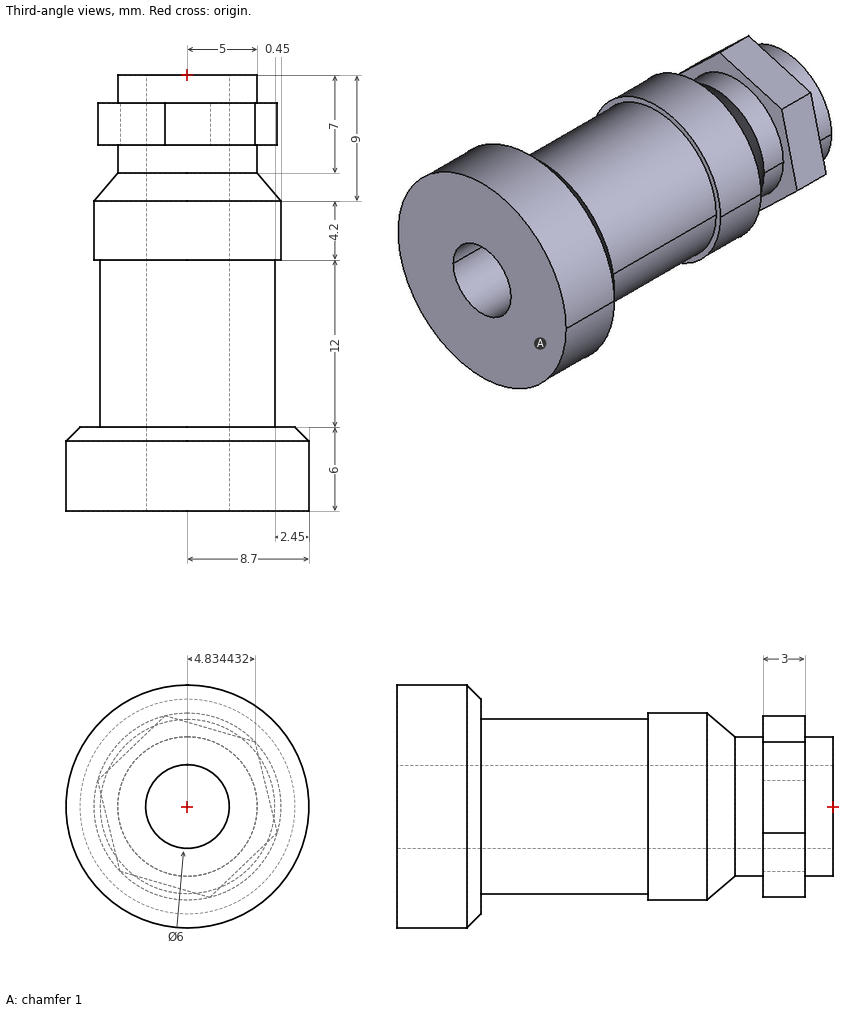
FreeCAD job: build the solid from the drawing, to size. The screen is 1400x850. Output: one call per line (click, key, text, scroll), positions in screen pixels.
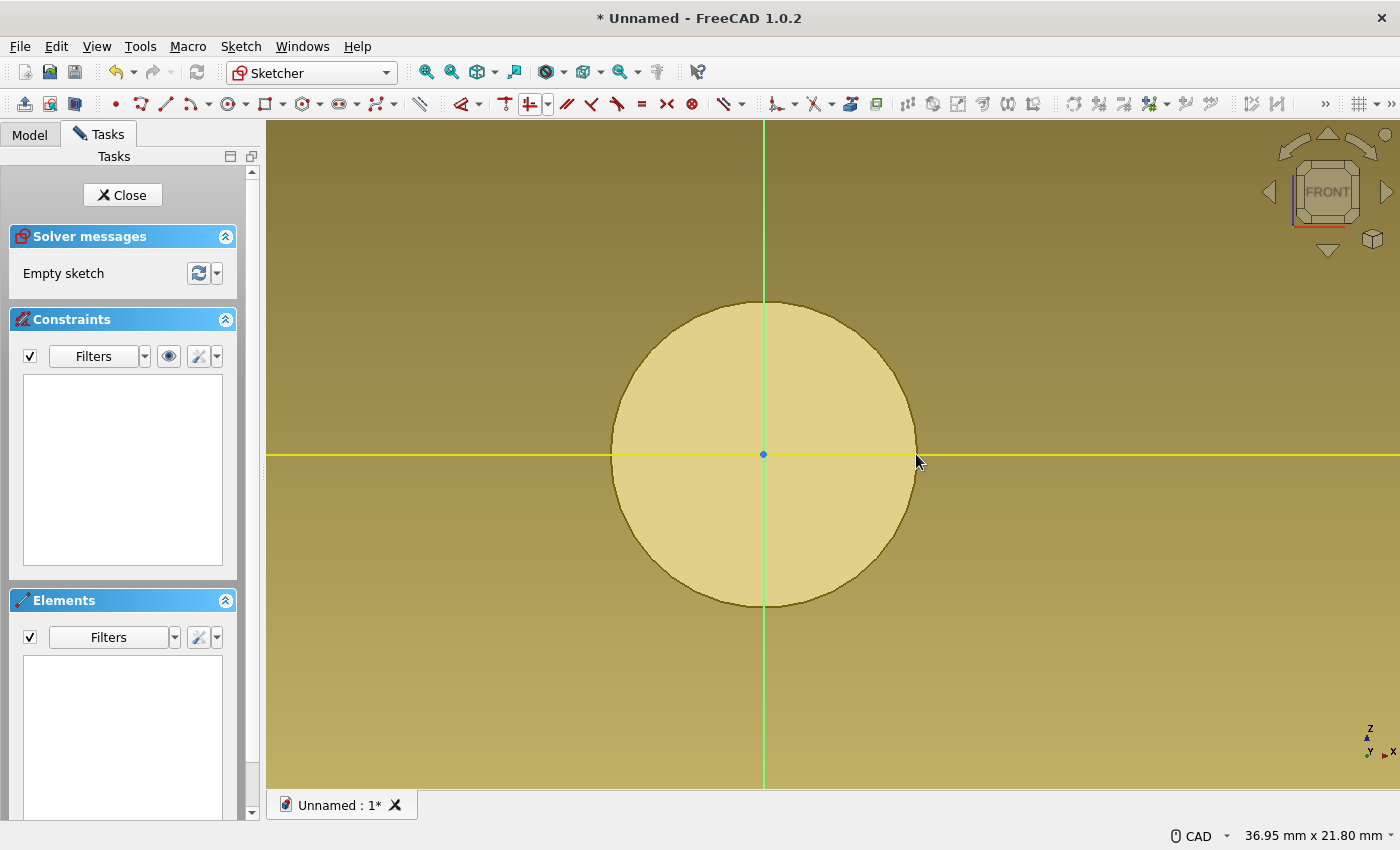
key(g)
key(p)
key(6)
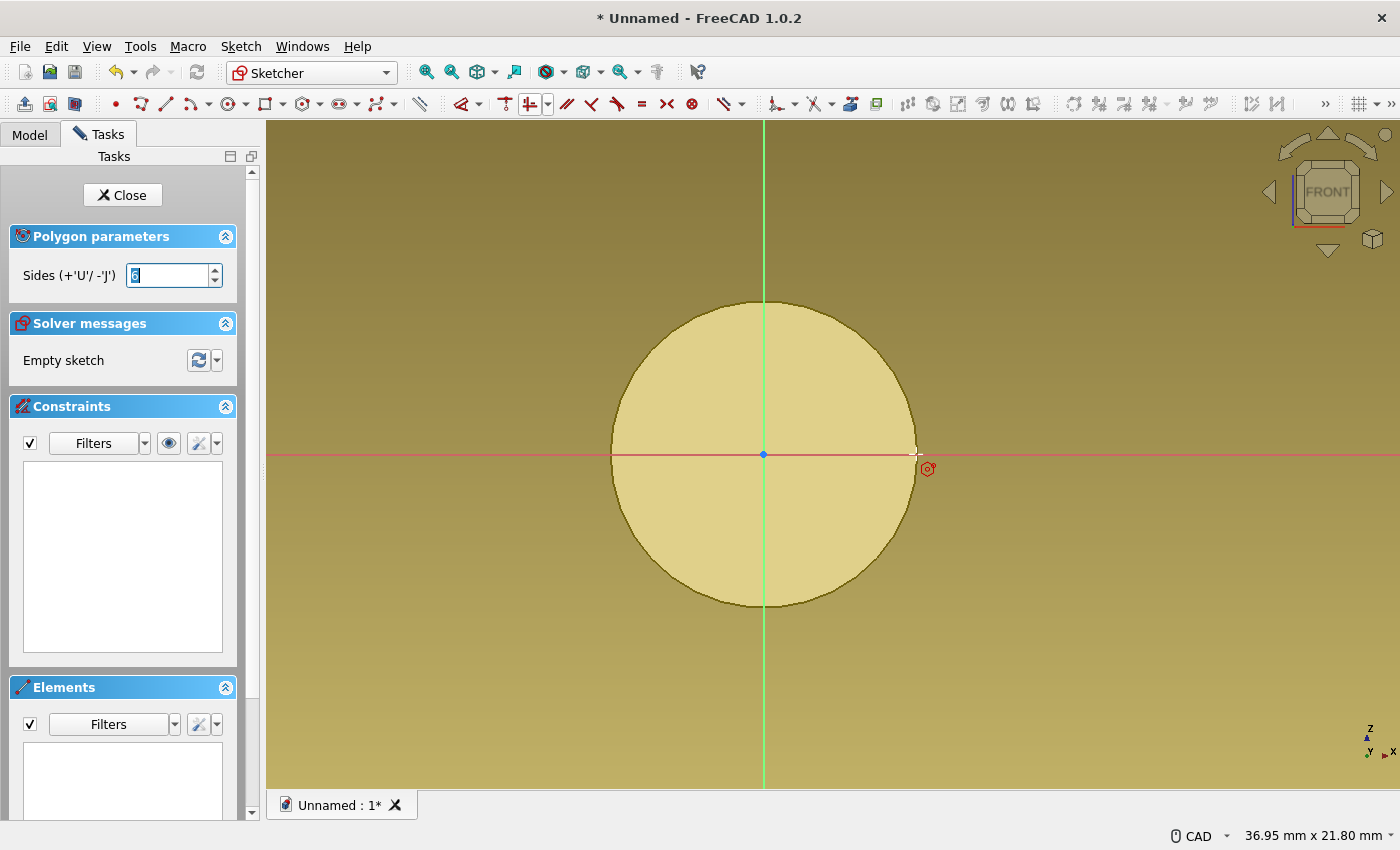
click(764, 454)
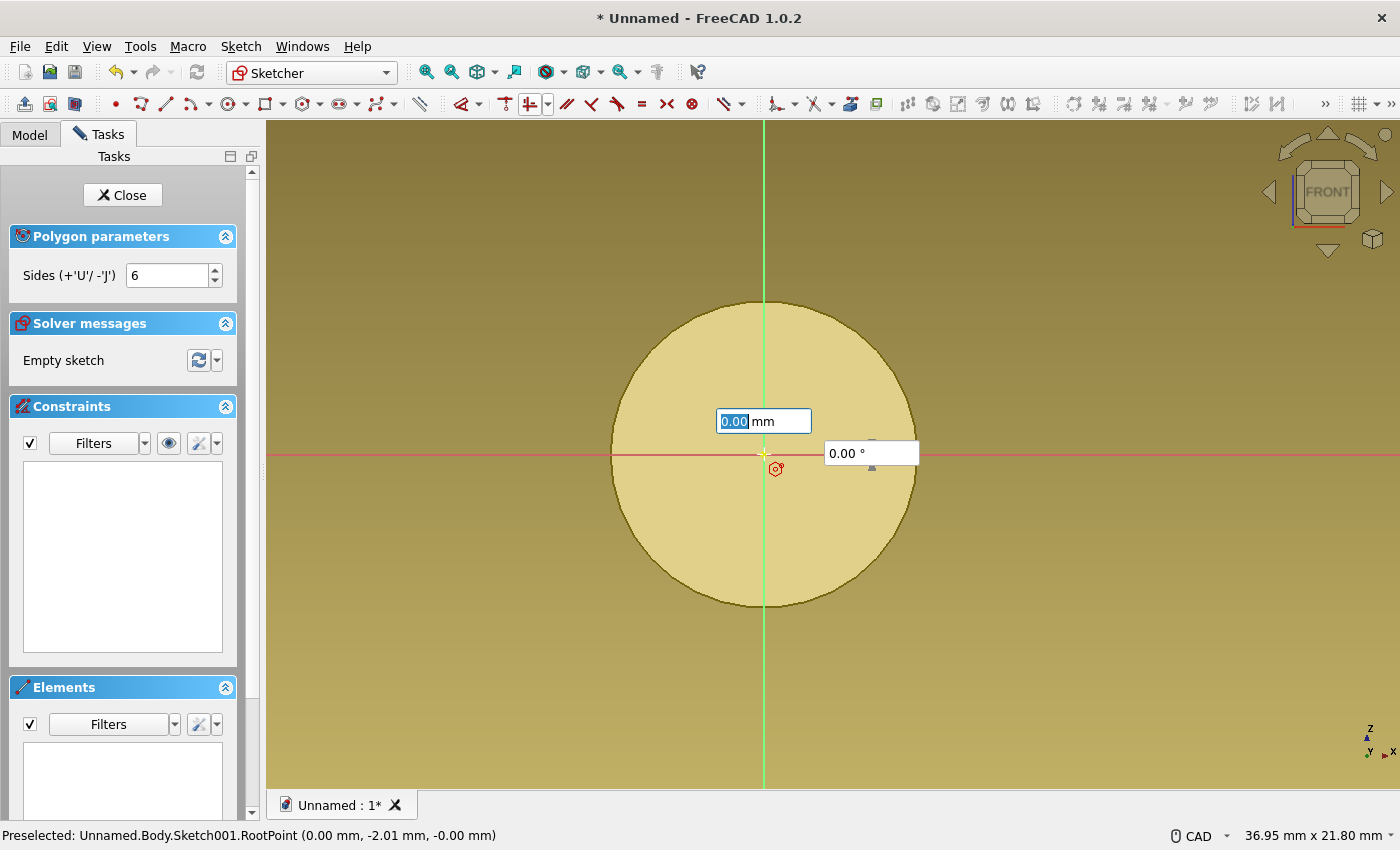
click(912, 312)
right_click(912, 312)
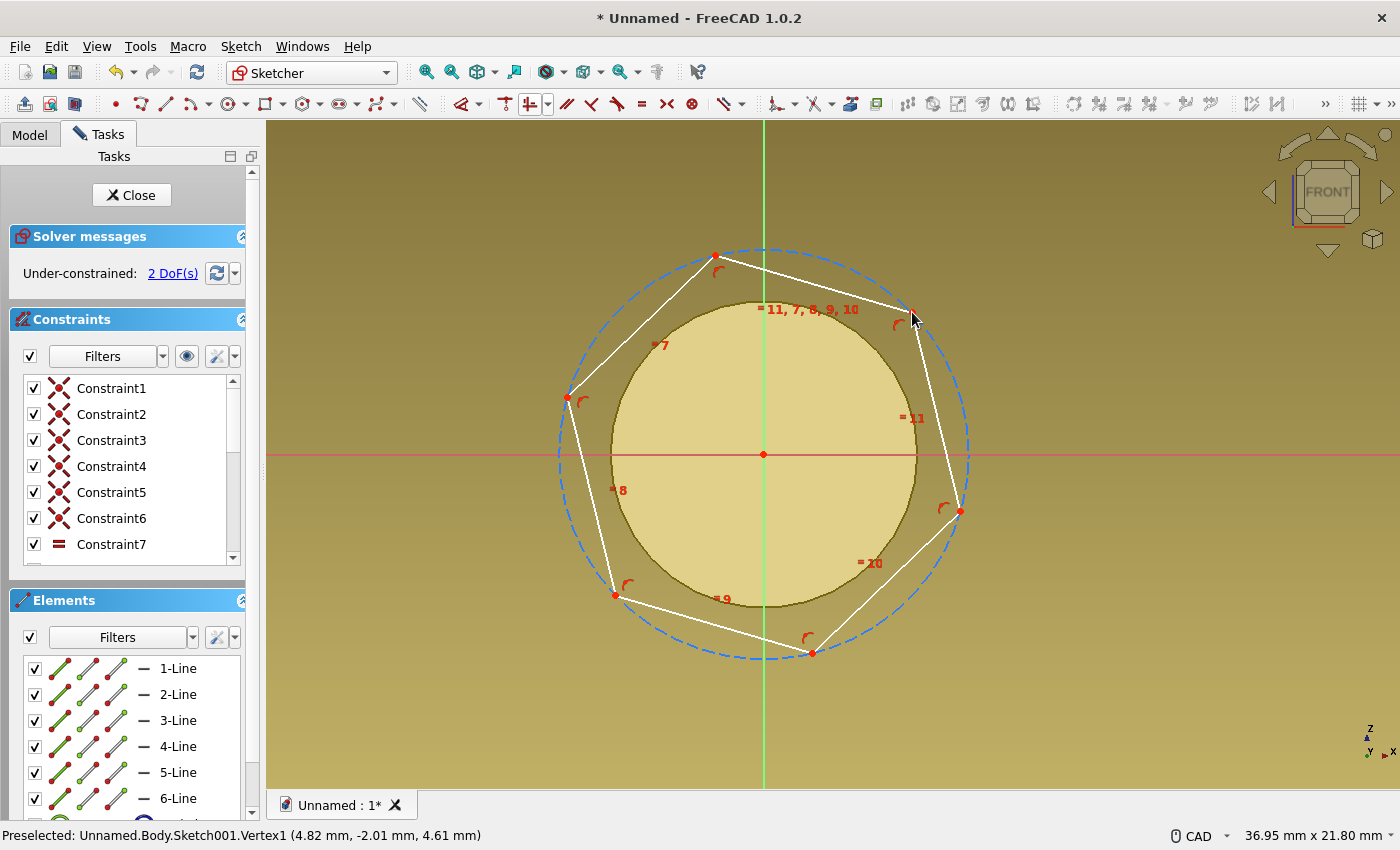
key(d)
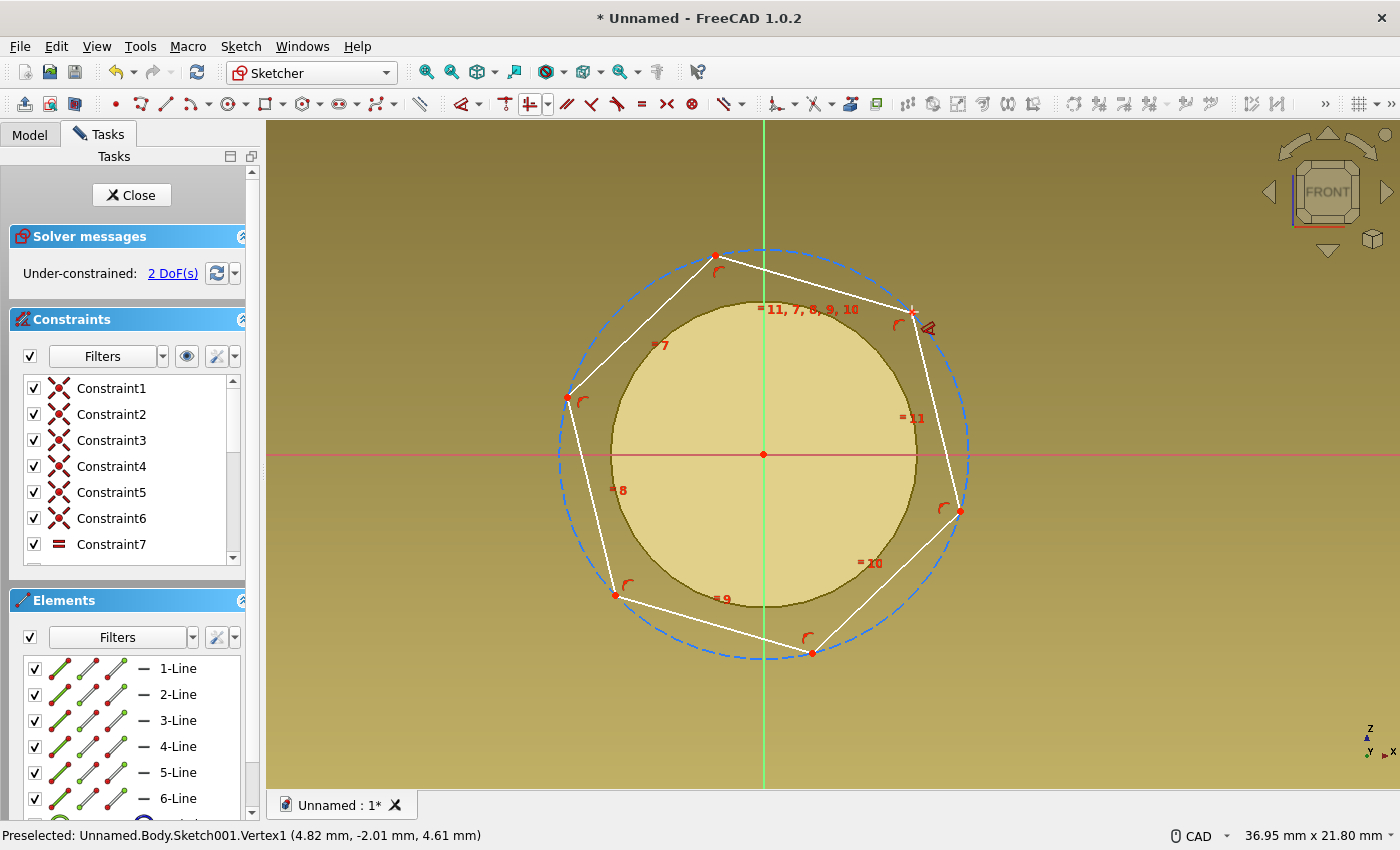
click(619, 310)
click(596, 287)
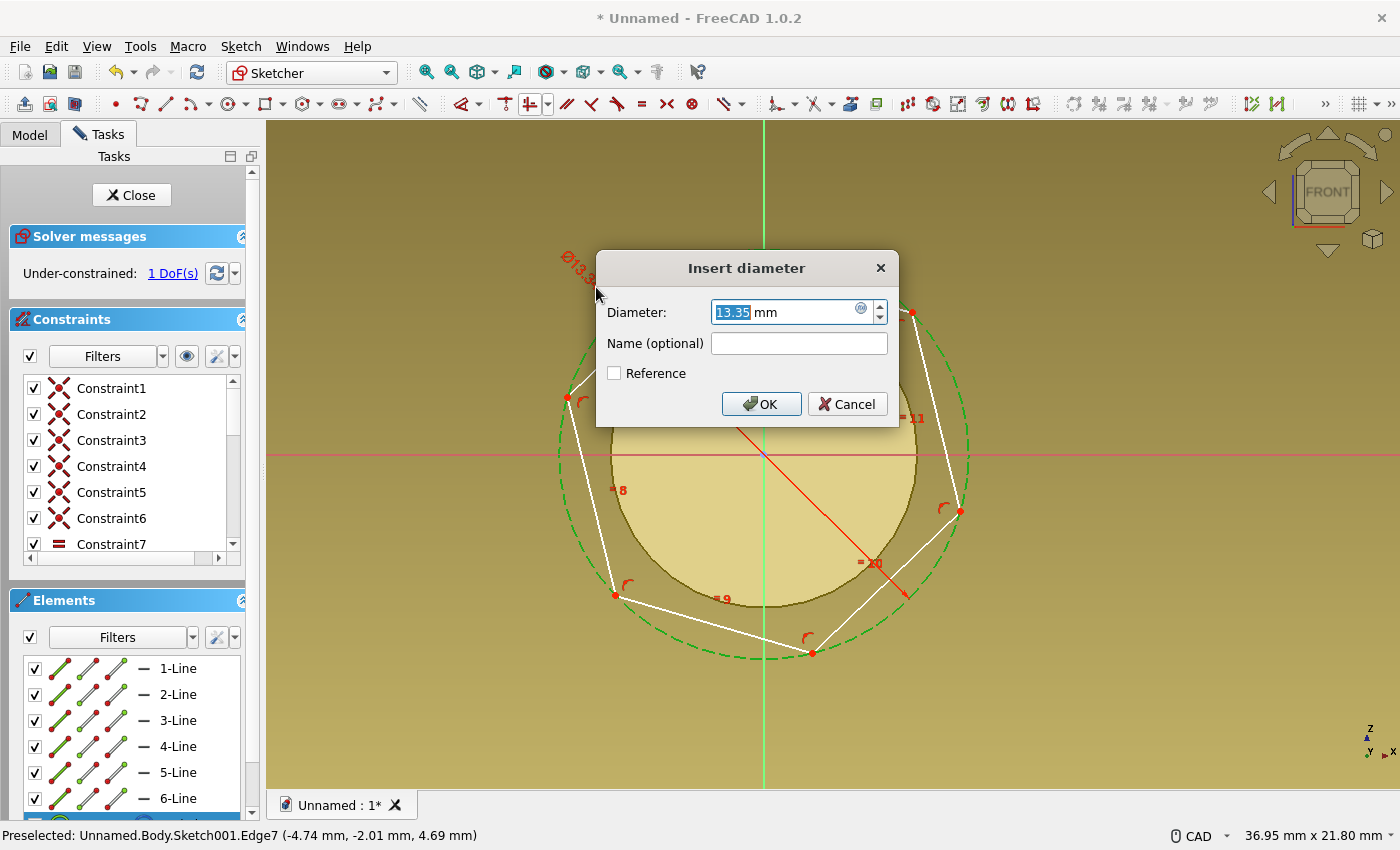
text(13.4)
key(Return)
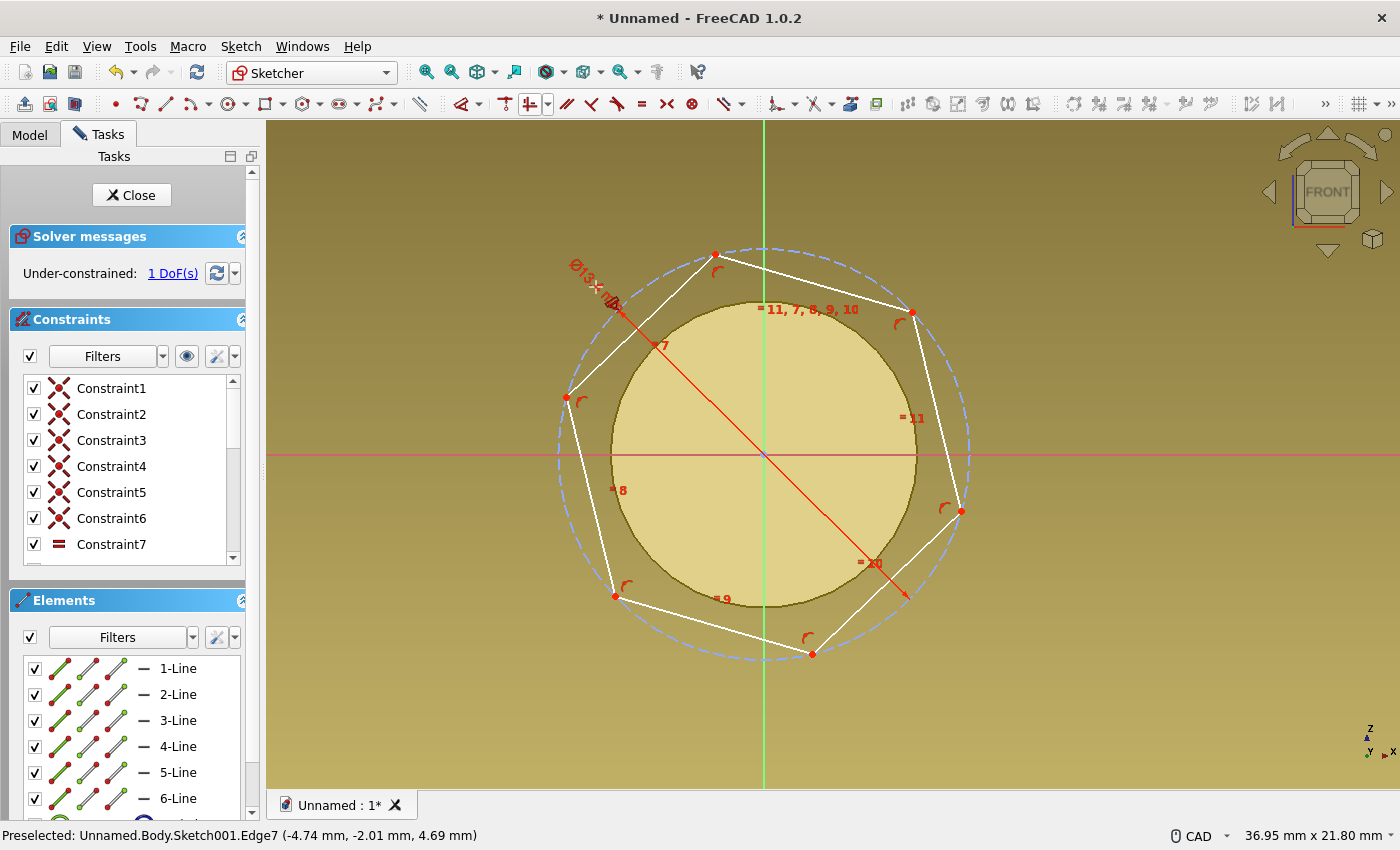
click(912, 312)
click(838, 488)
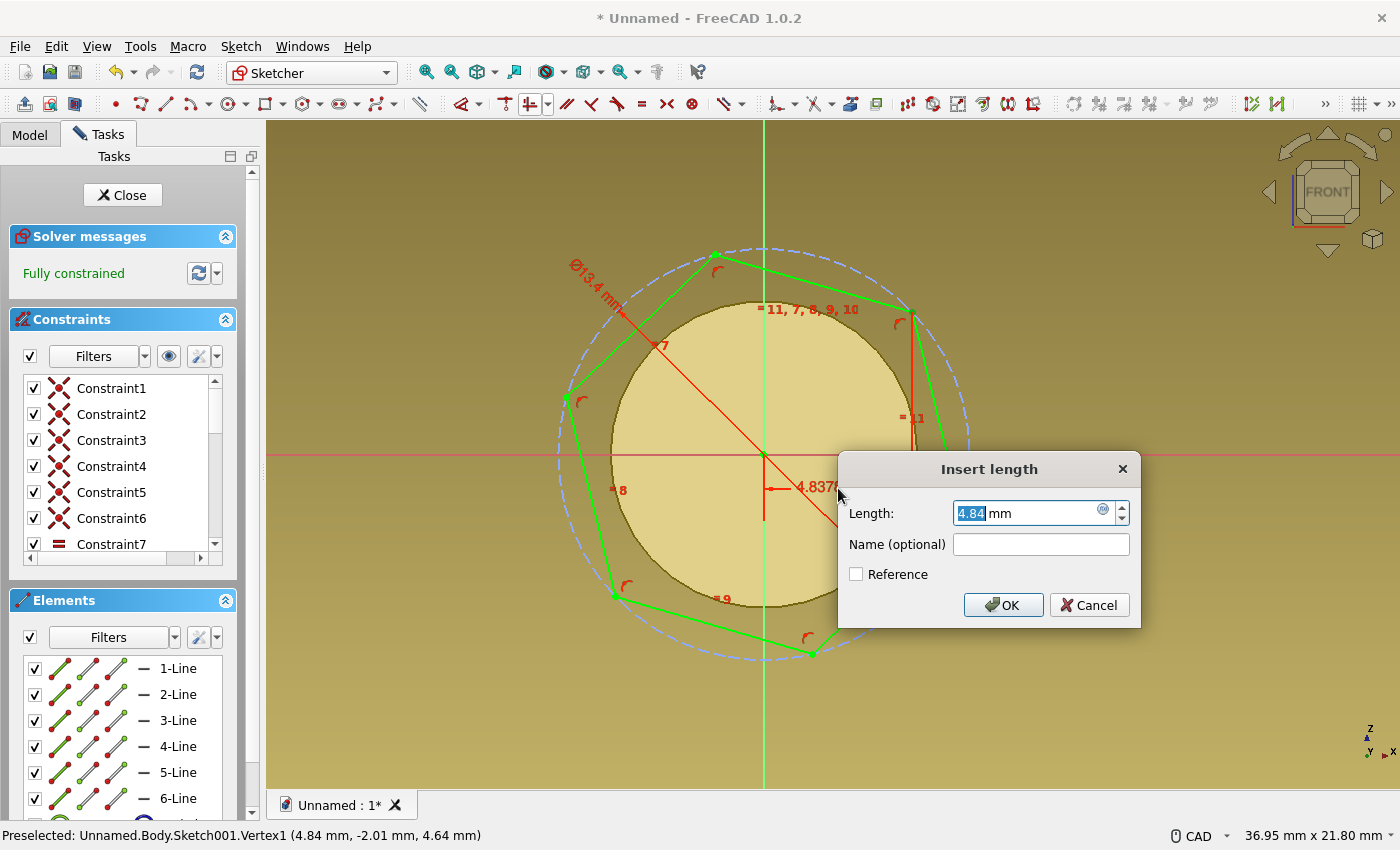
text(4.834432)
key(Return)
key(Escape)